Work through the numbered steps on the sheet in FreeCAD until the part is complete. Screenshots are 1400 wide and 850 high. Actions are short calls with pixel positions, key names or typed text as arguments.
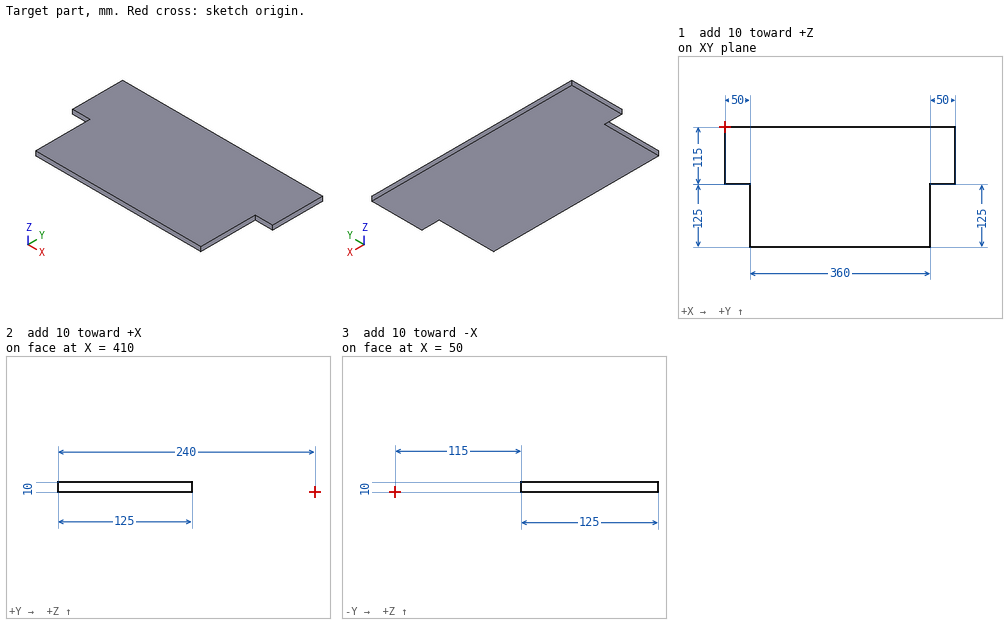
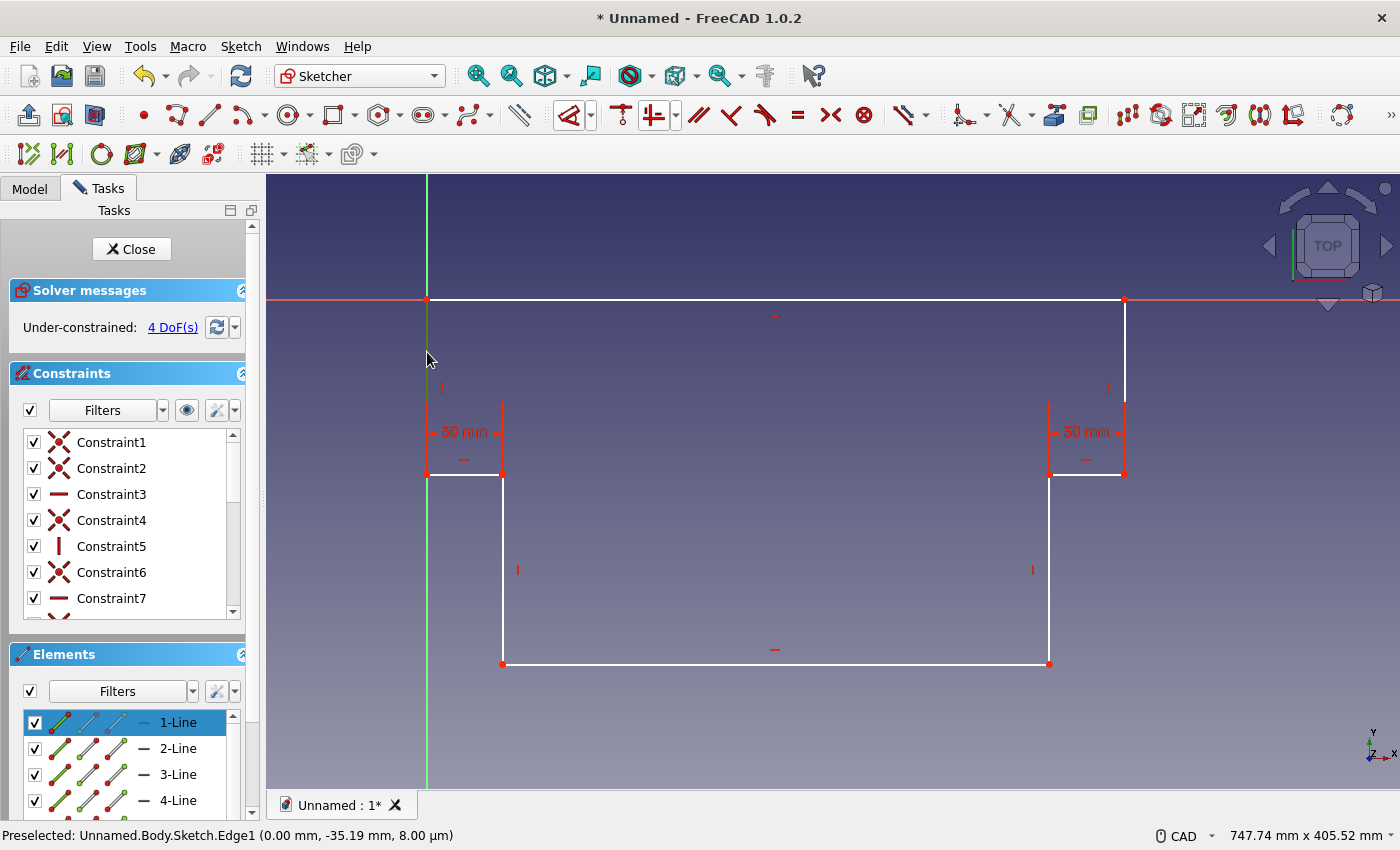
key(i)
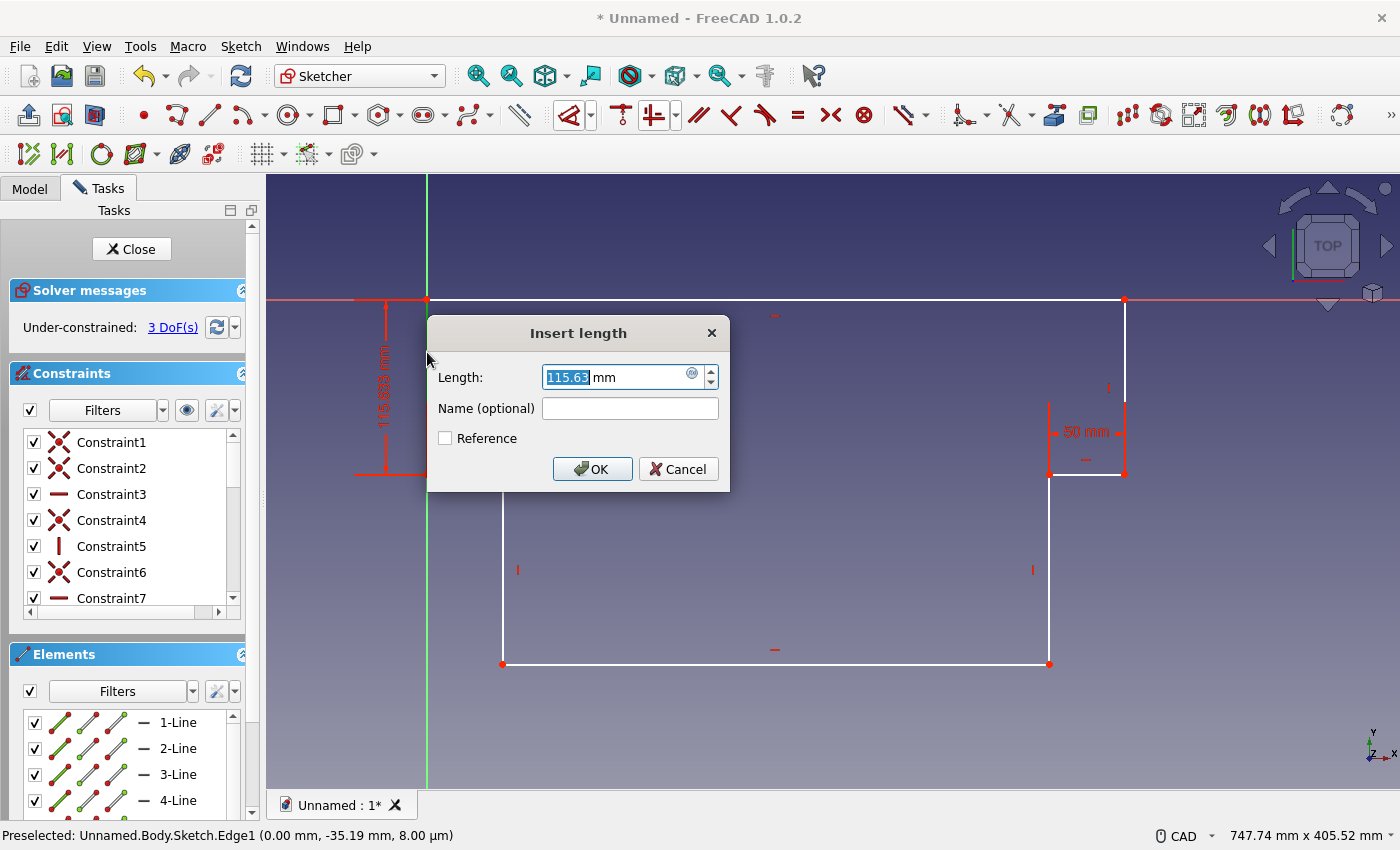
text(115)
key(Return)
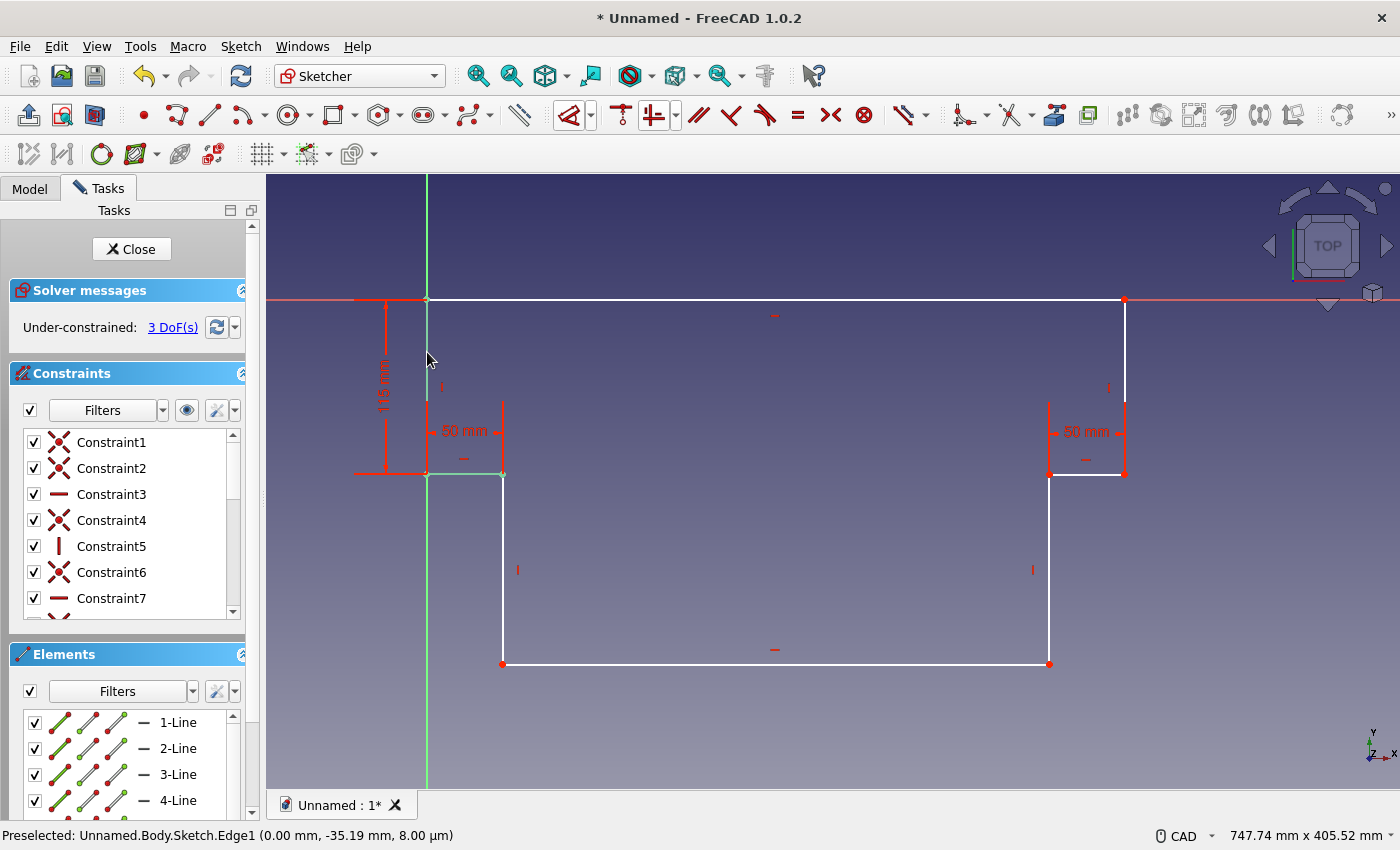
click(503, 531)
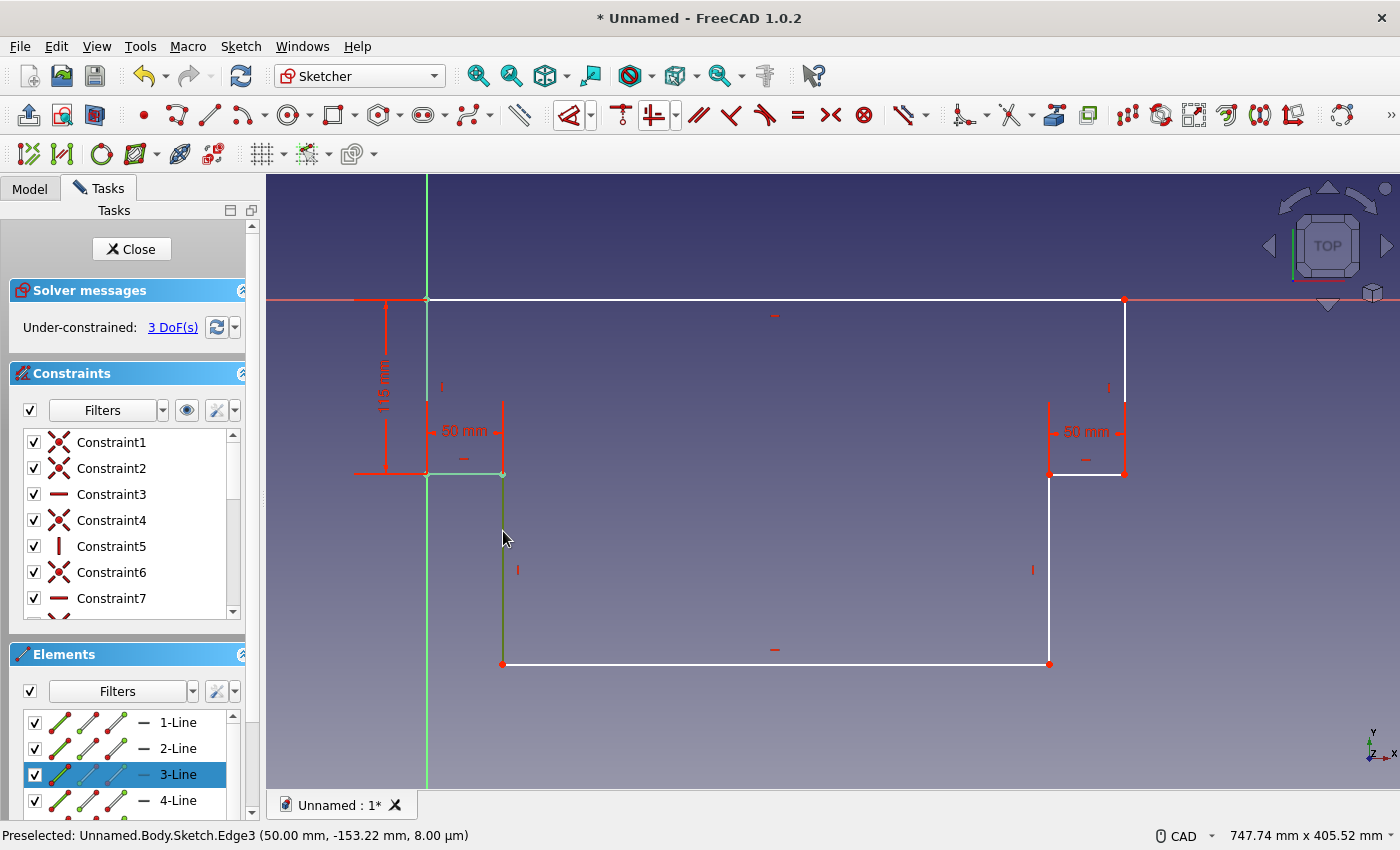
click(590, 116)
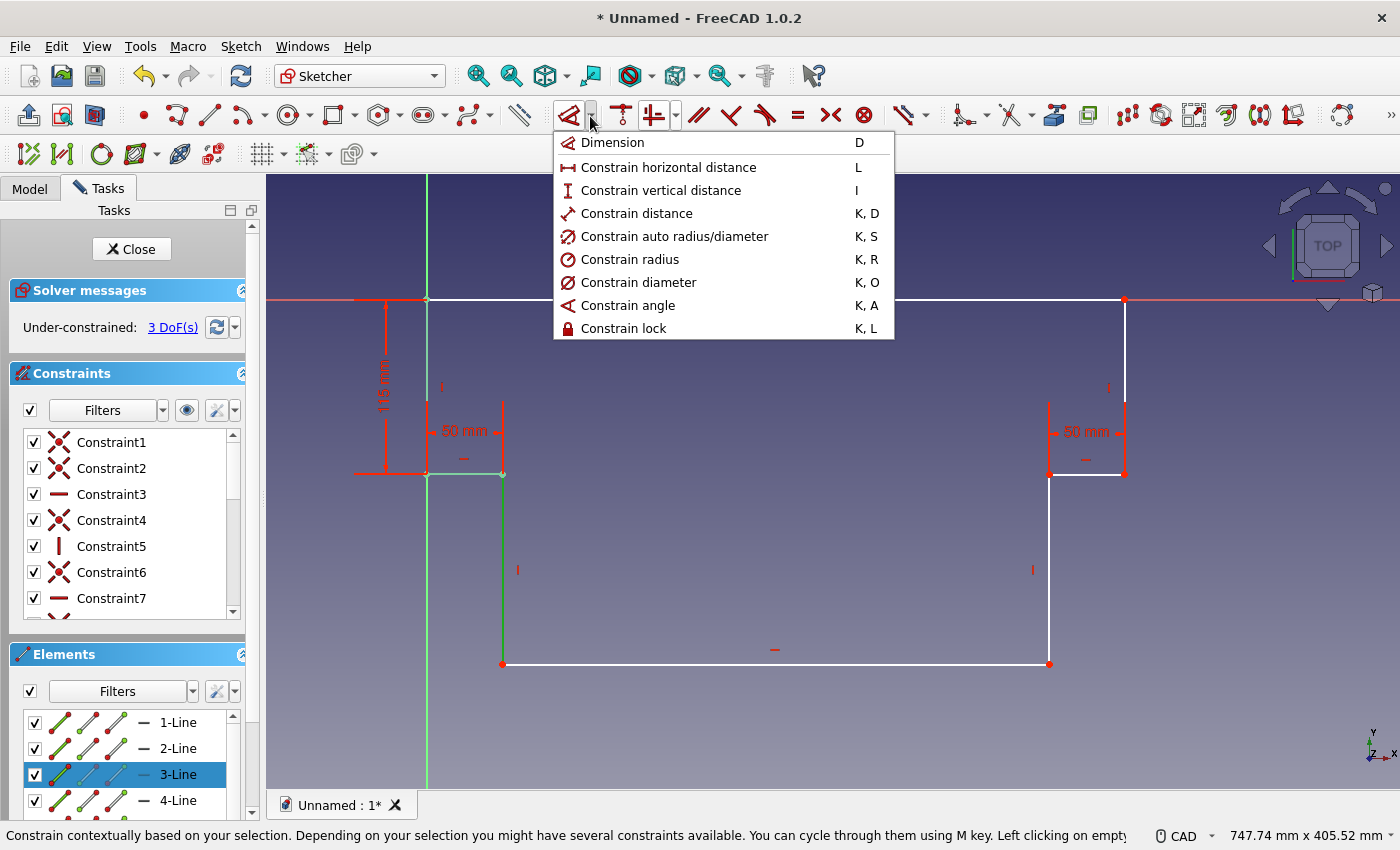
click(724, 190)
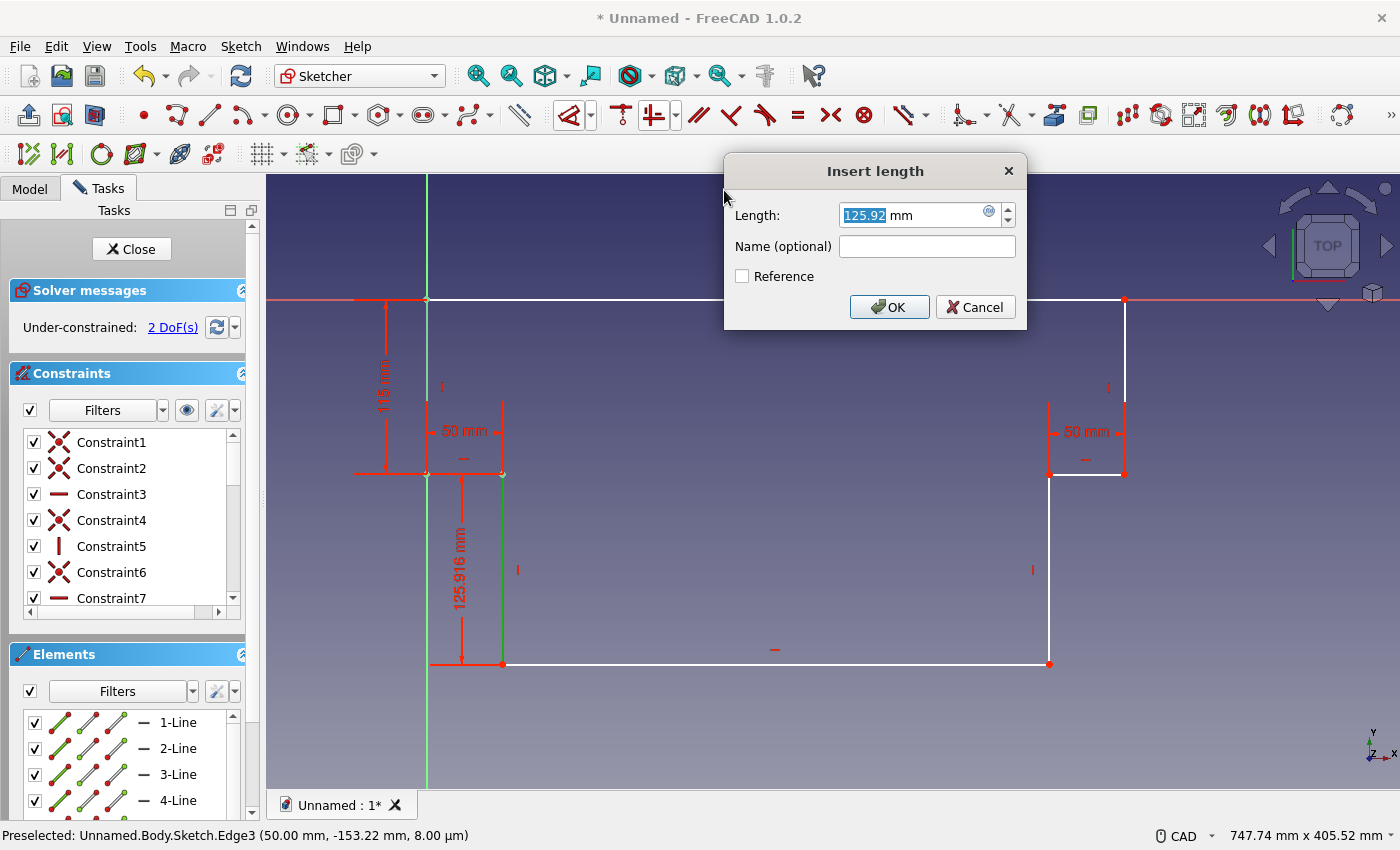
text(125)
key(Return)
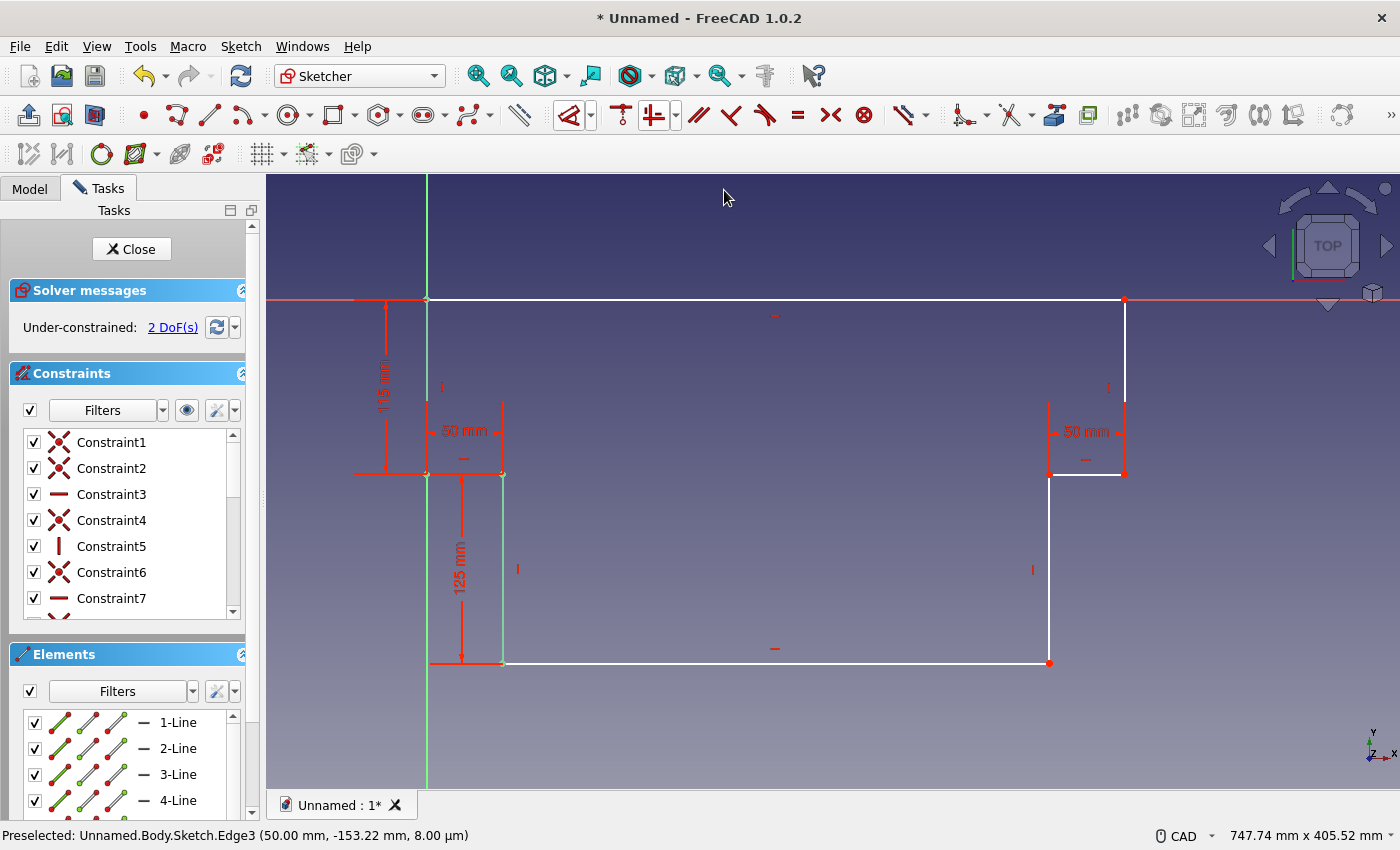
click(667, 664)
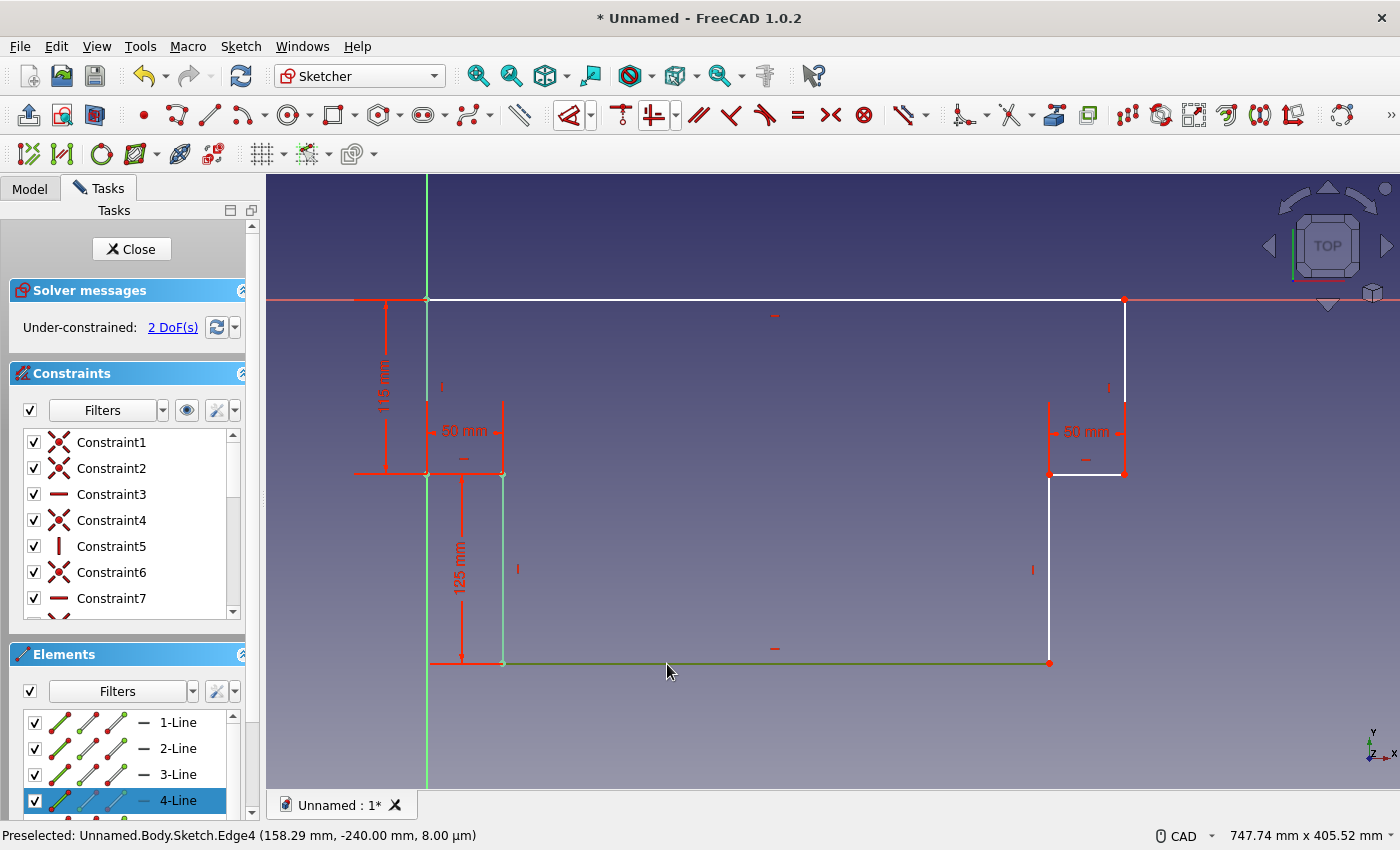
key(l)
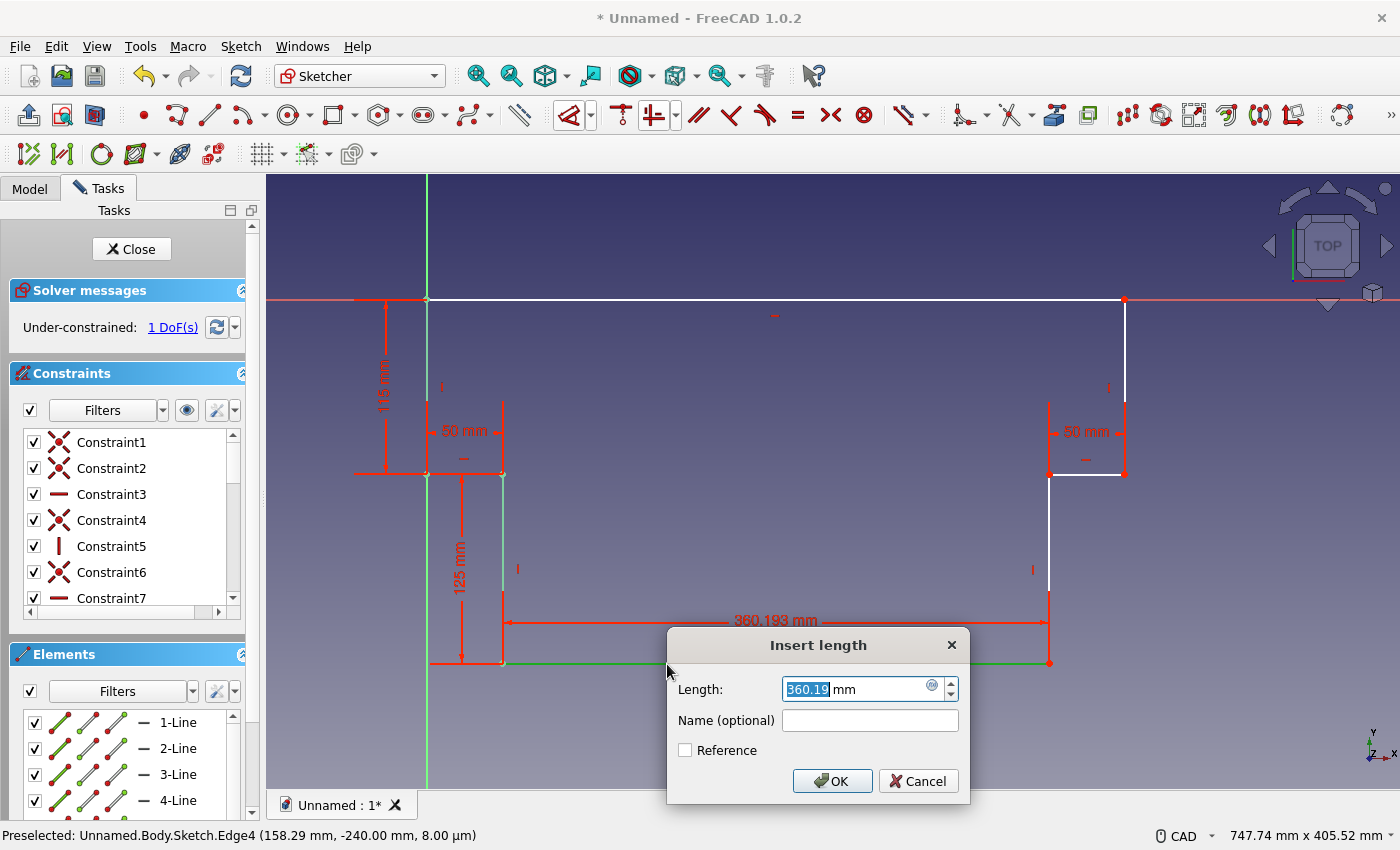
text(360)
key(Return)